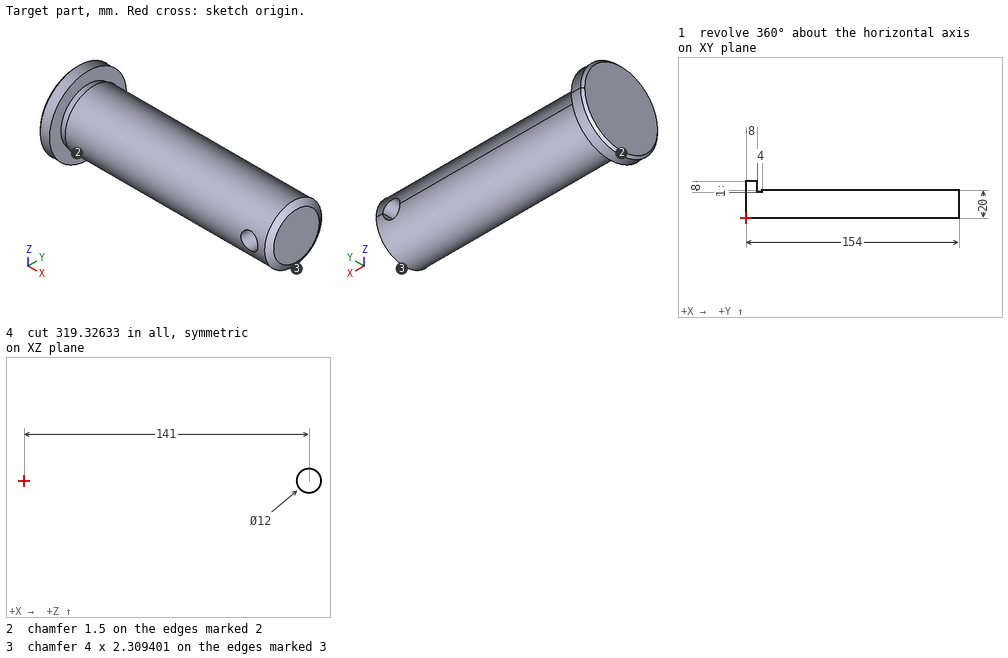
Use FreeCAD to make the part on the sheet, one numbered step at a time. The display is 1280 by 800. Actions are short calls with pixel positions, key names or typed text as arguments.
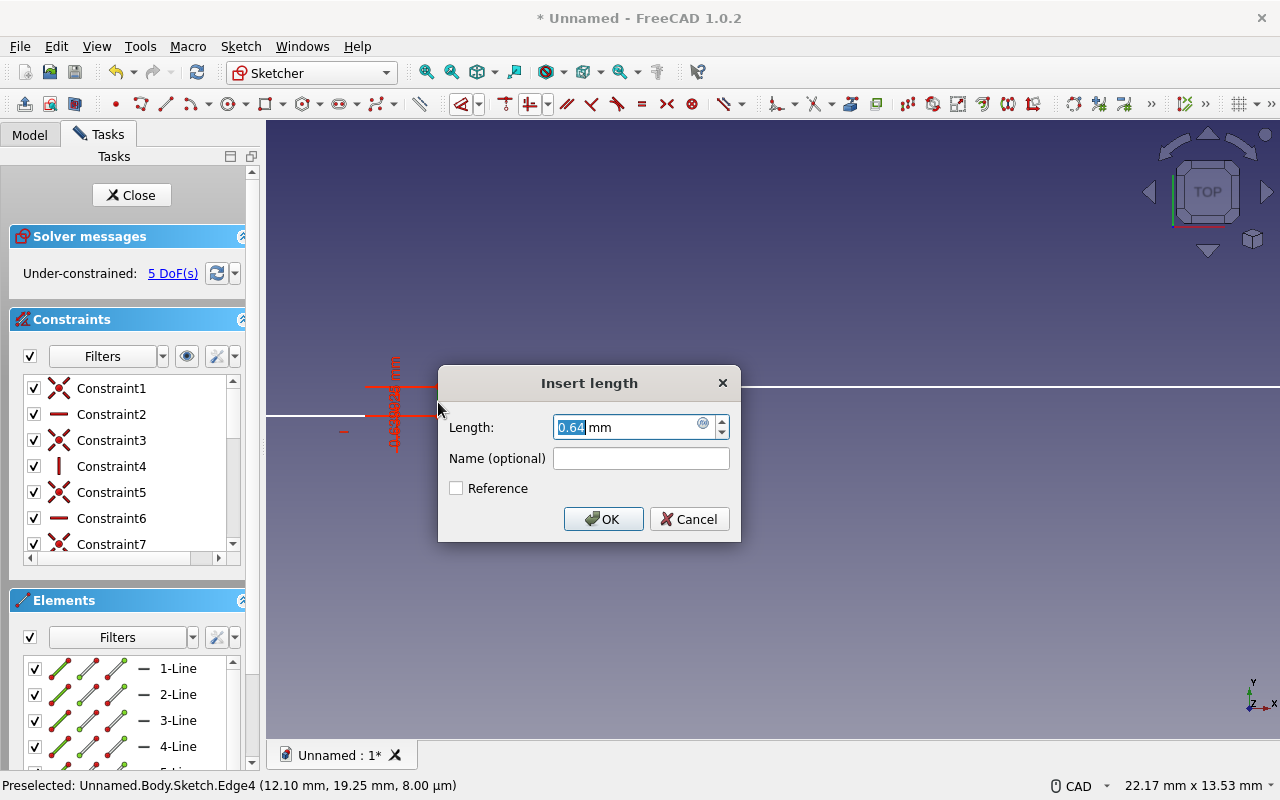
text(1)
key(Return)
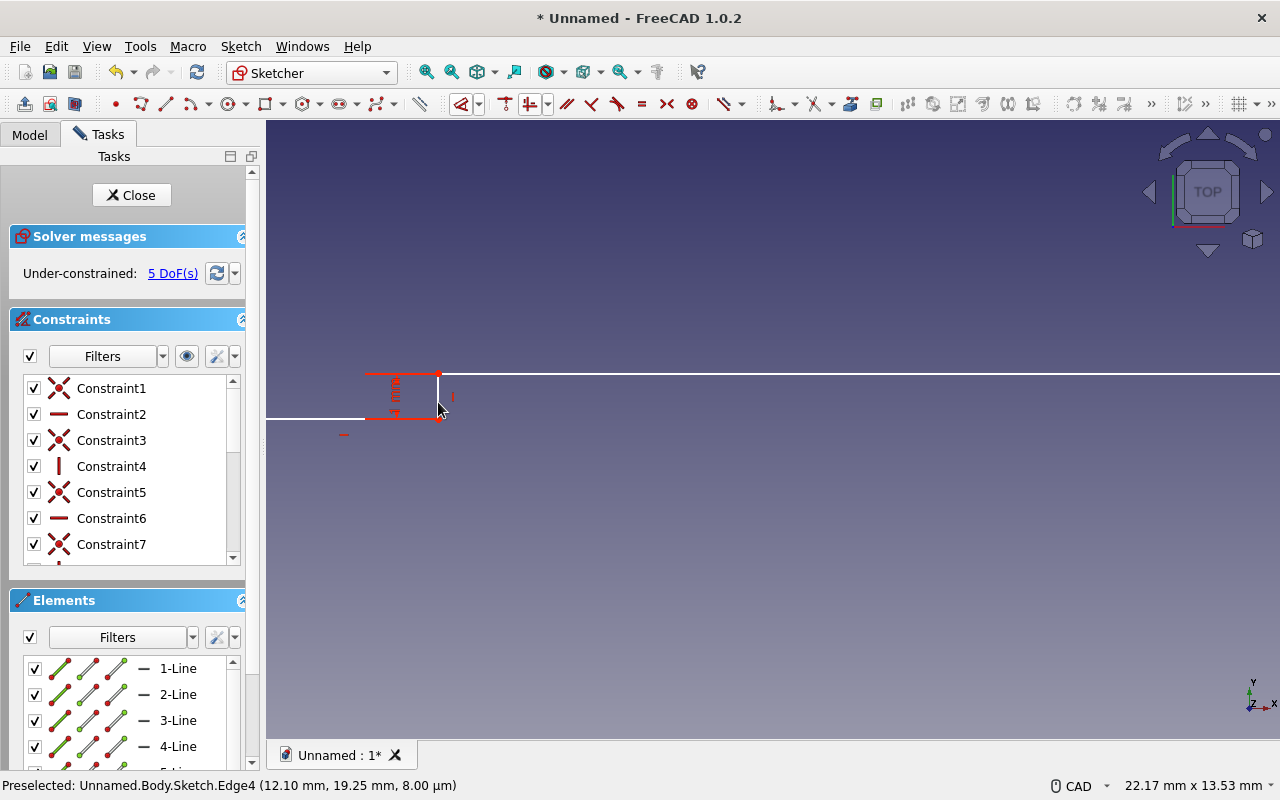
scroll(435, 406, down, 12)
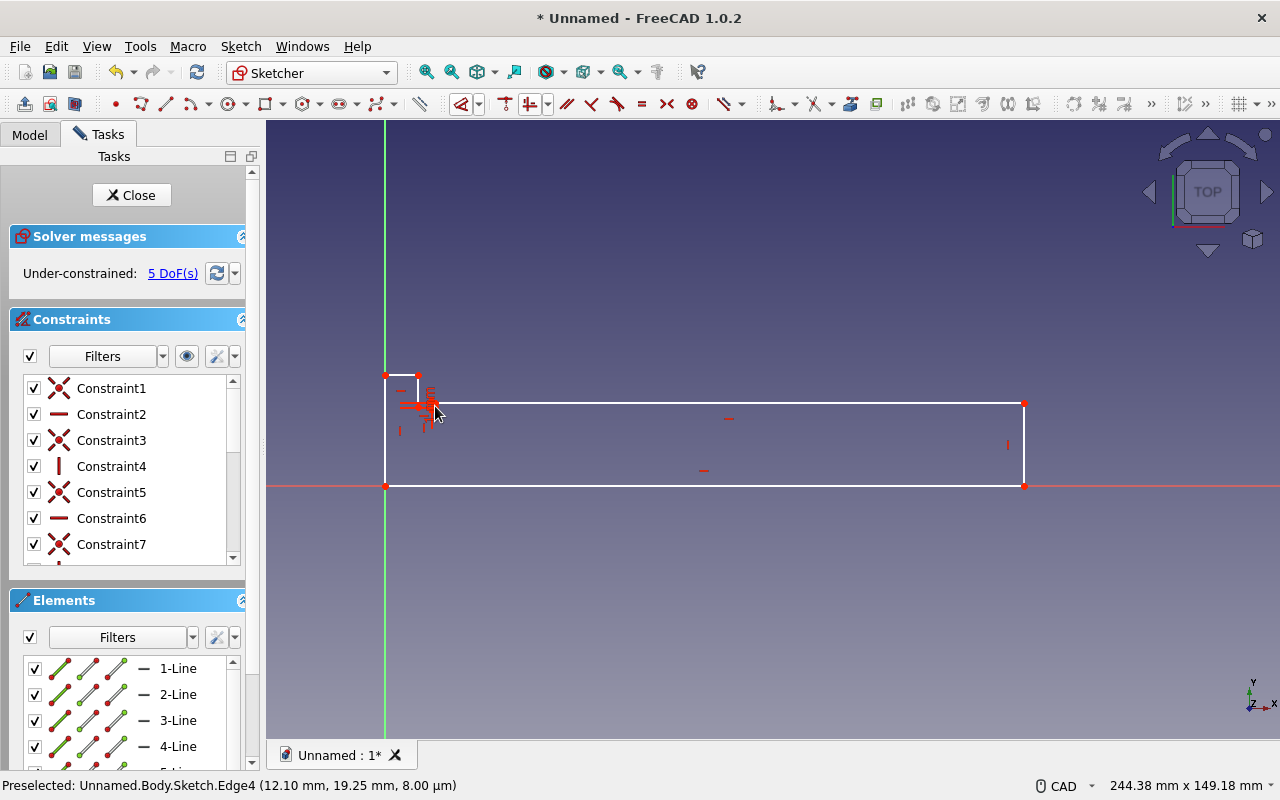
scroll(430, 408, up, 5)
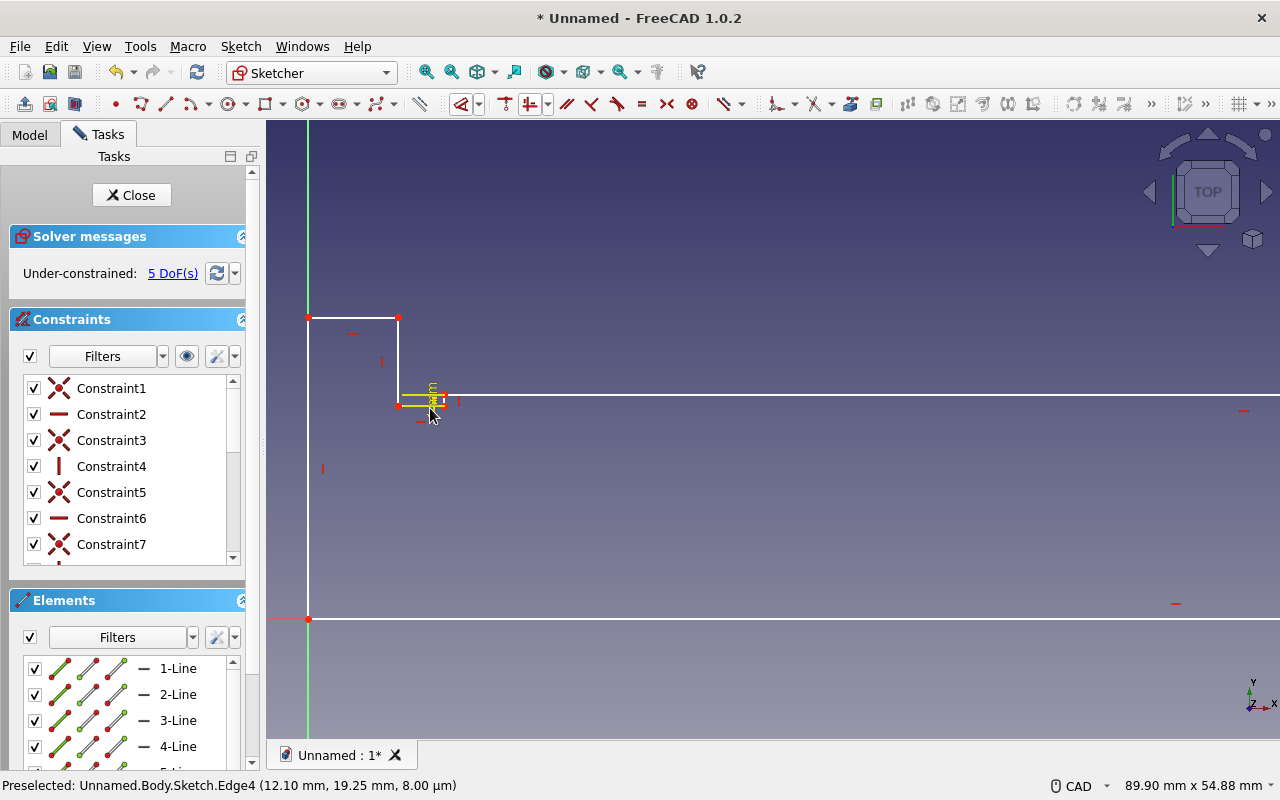
click(412, 406)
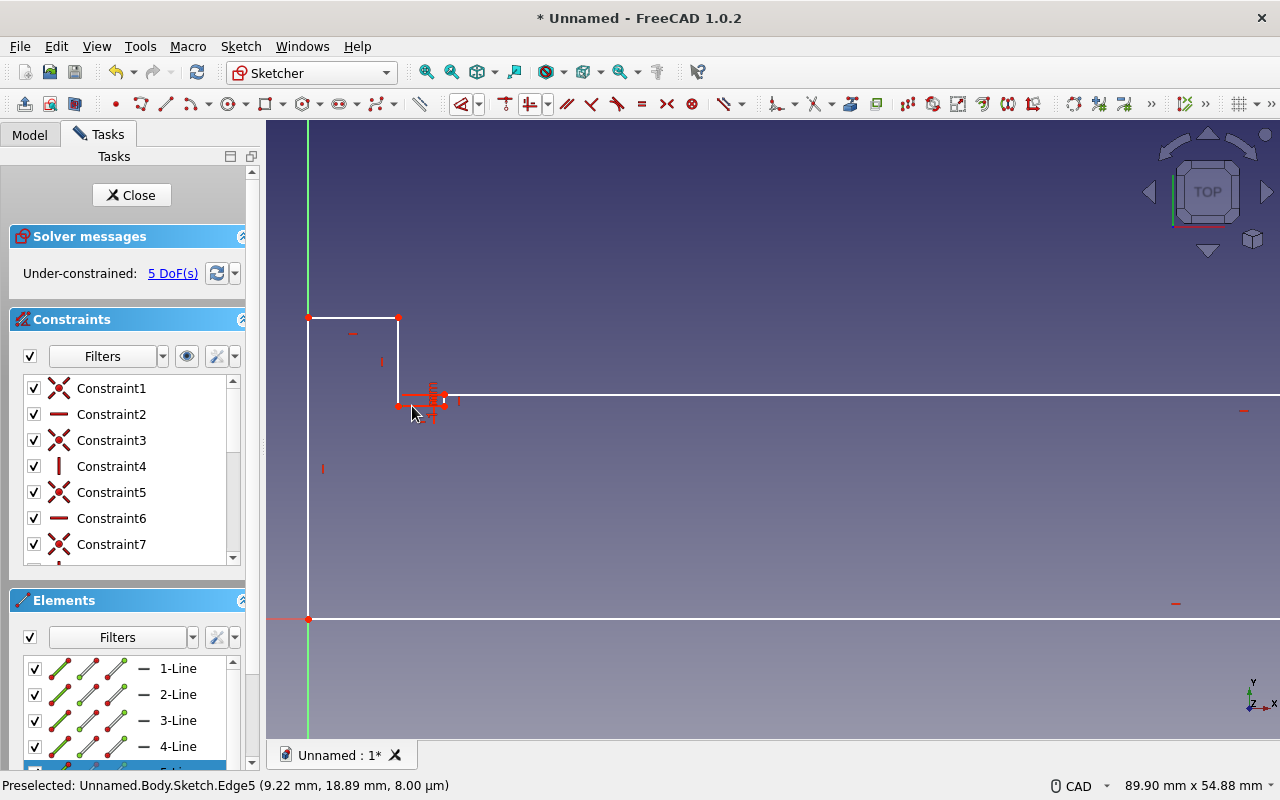
click(478, 104)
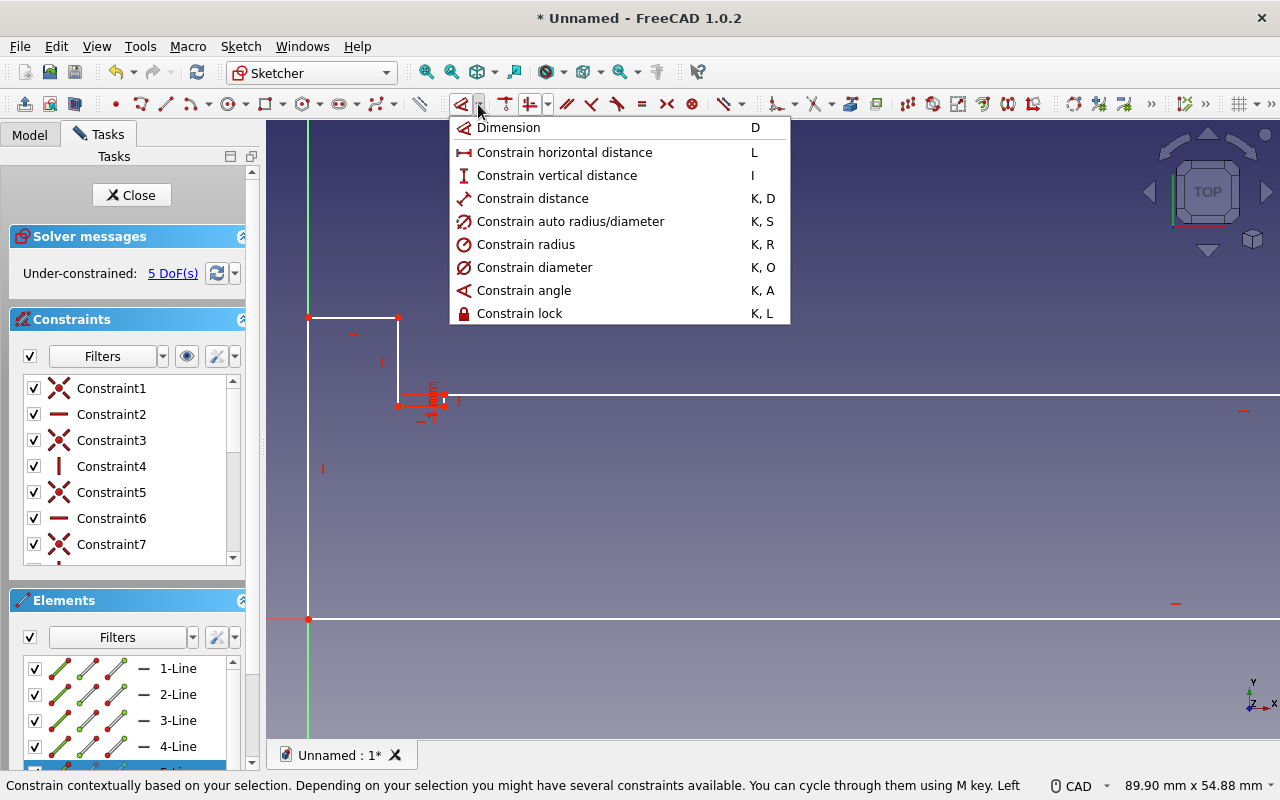
click(620, 152)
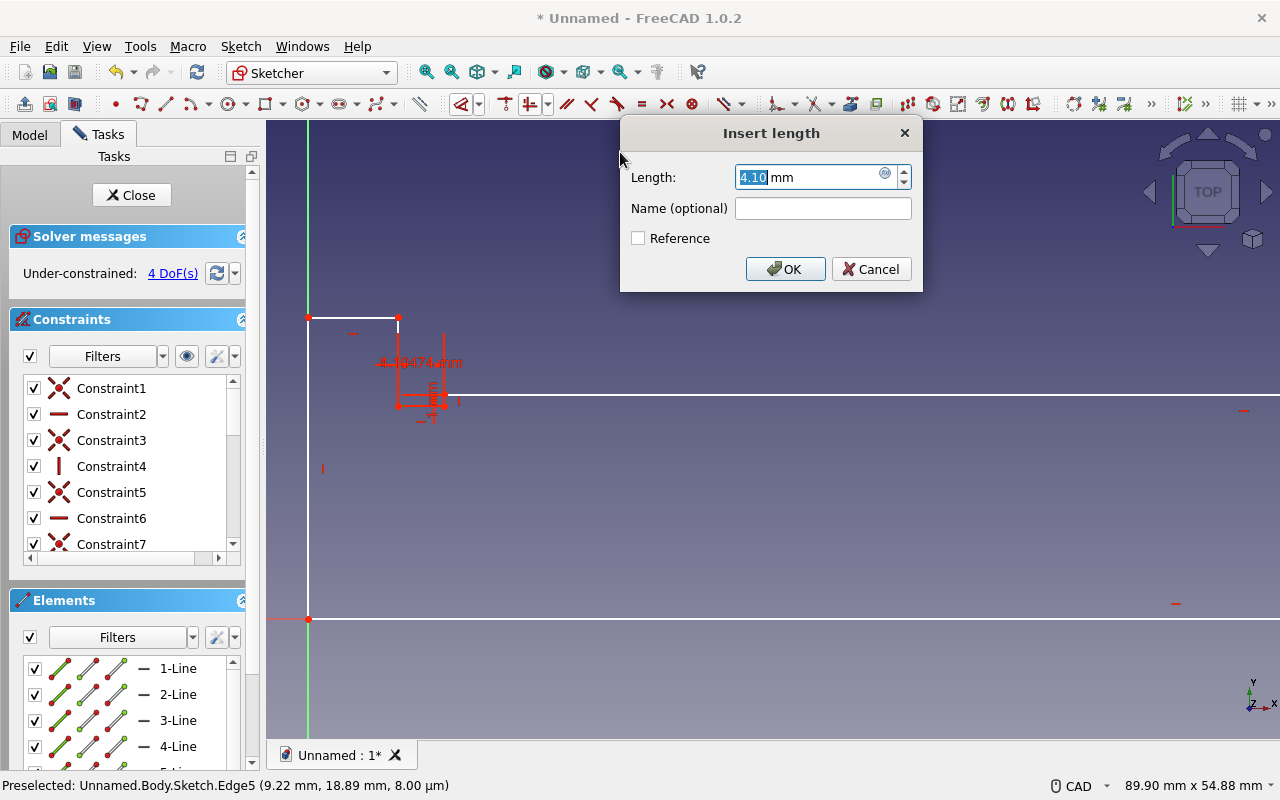
text(4)
key(Return)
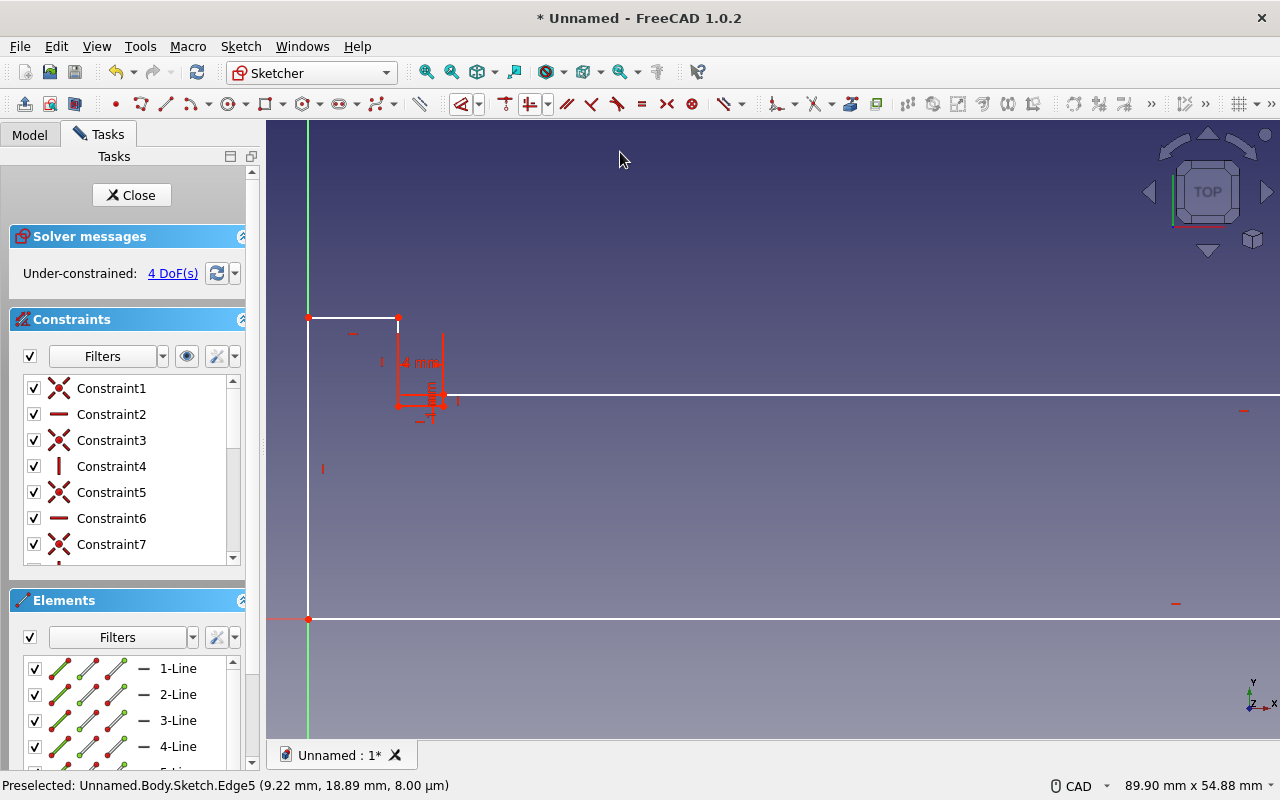
click(398, 380)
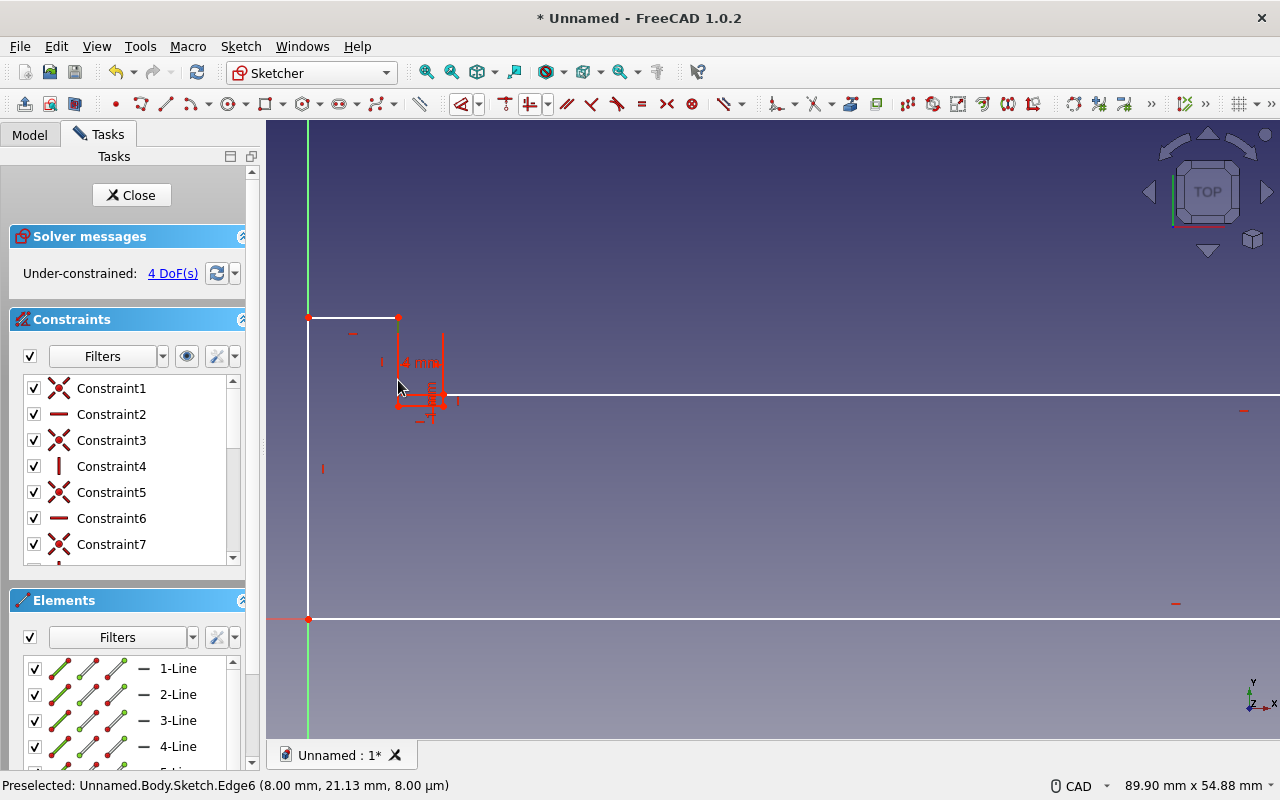
key(i)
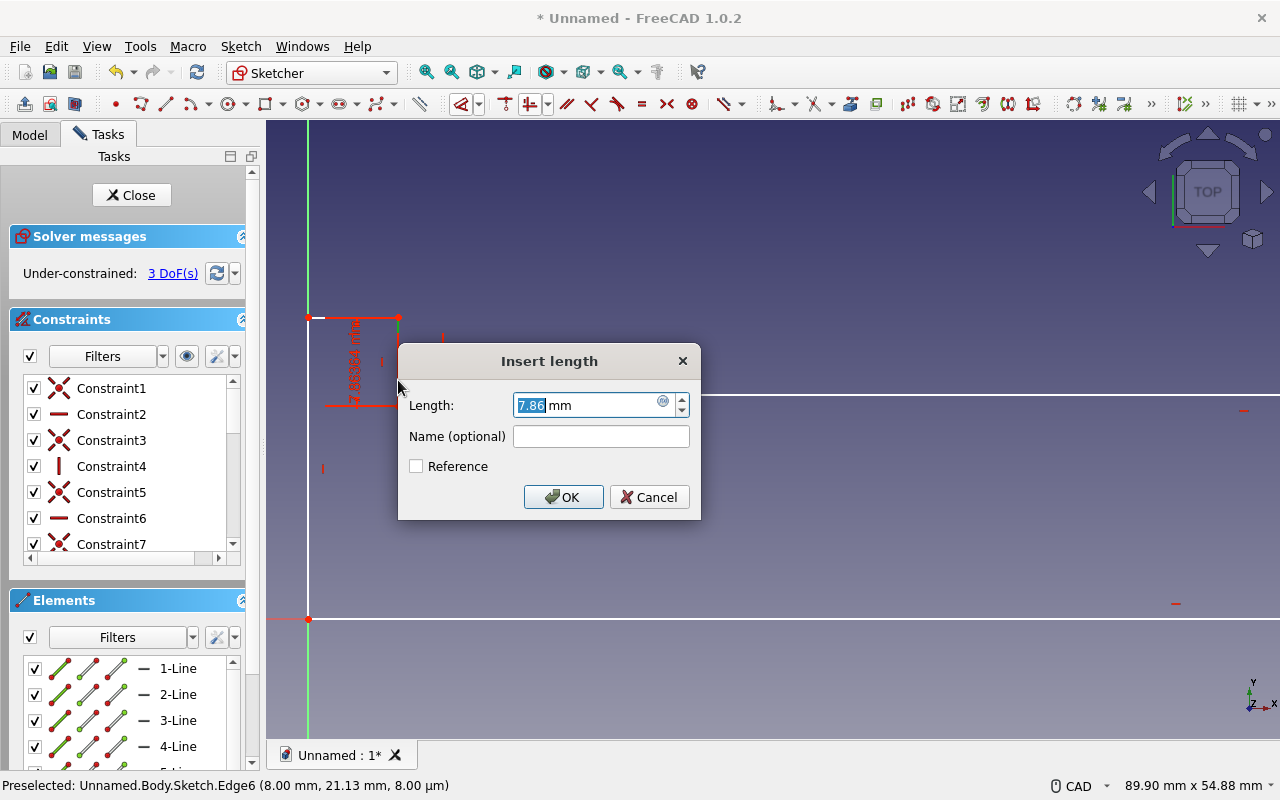
text(8)
key(Return)